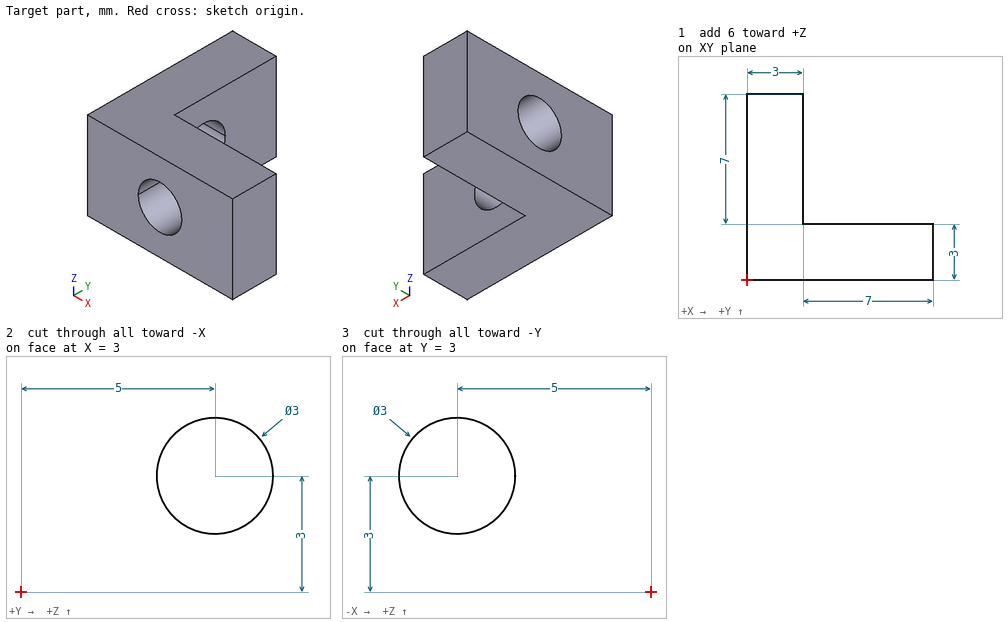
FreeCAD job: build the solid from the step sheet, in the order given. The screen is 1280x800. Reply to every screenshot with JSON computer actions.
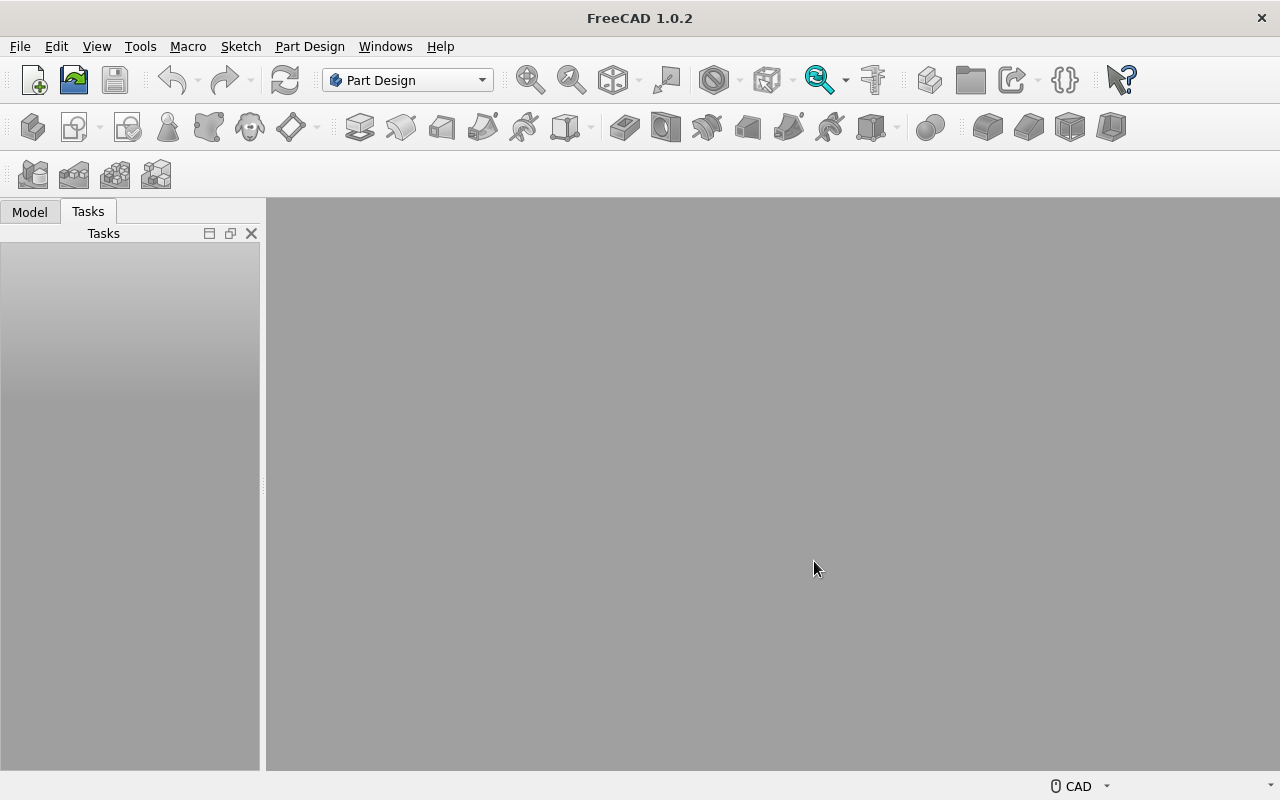
{"action": "left_click", "coordinate": [33, 80]}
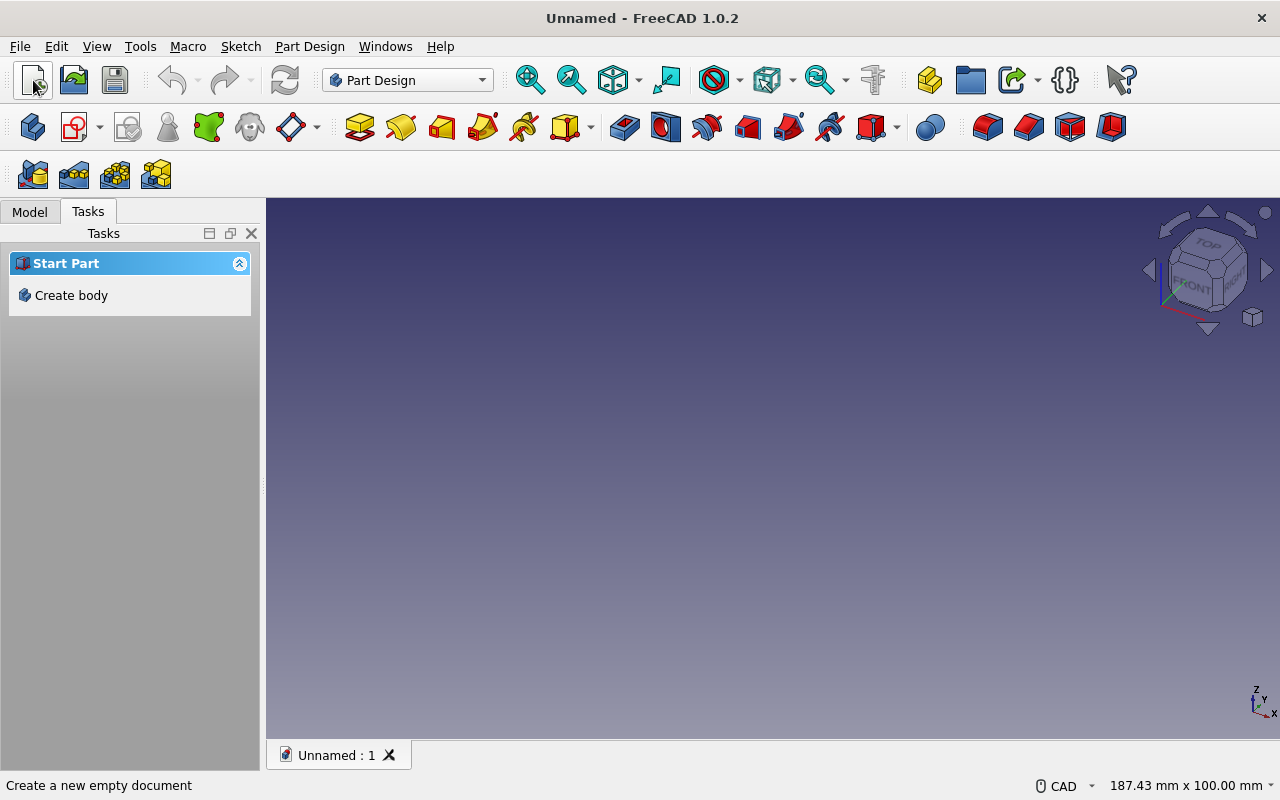
{"action": "left_click", "coordinate": [74, 128]}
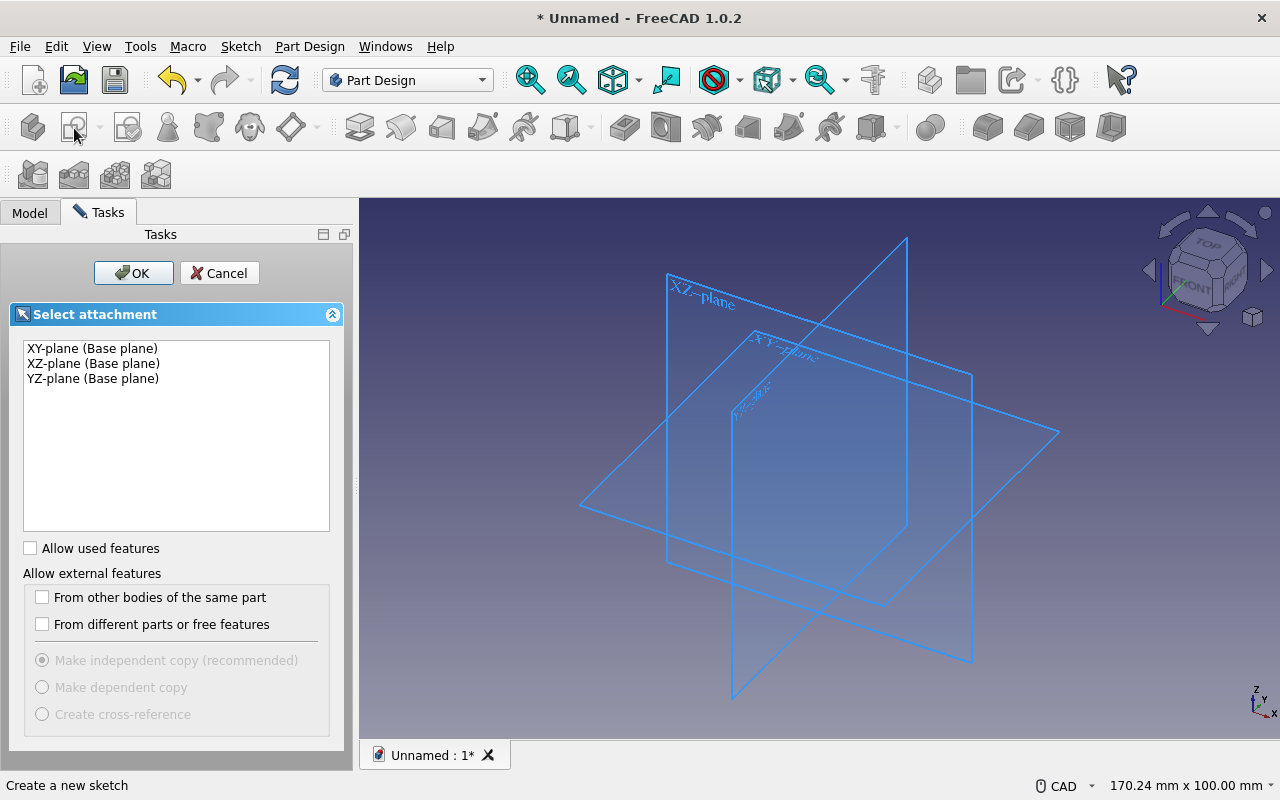
{"action": "left_click", "coordinate": [84, 348]}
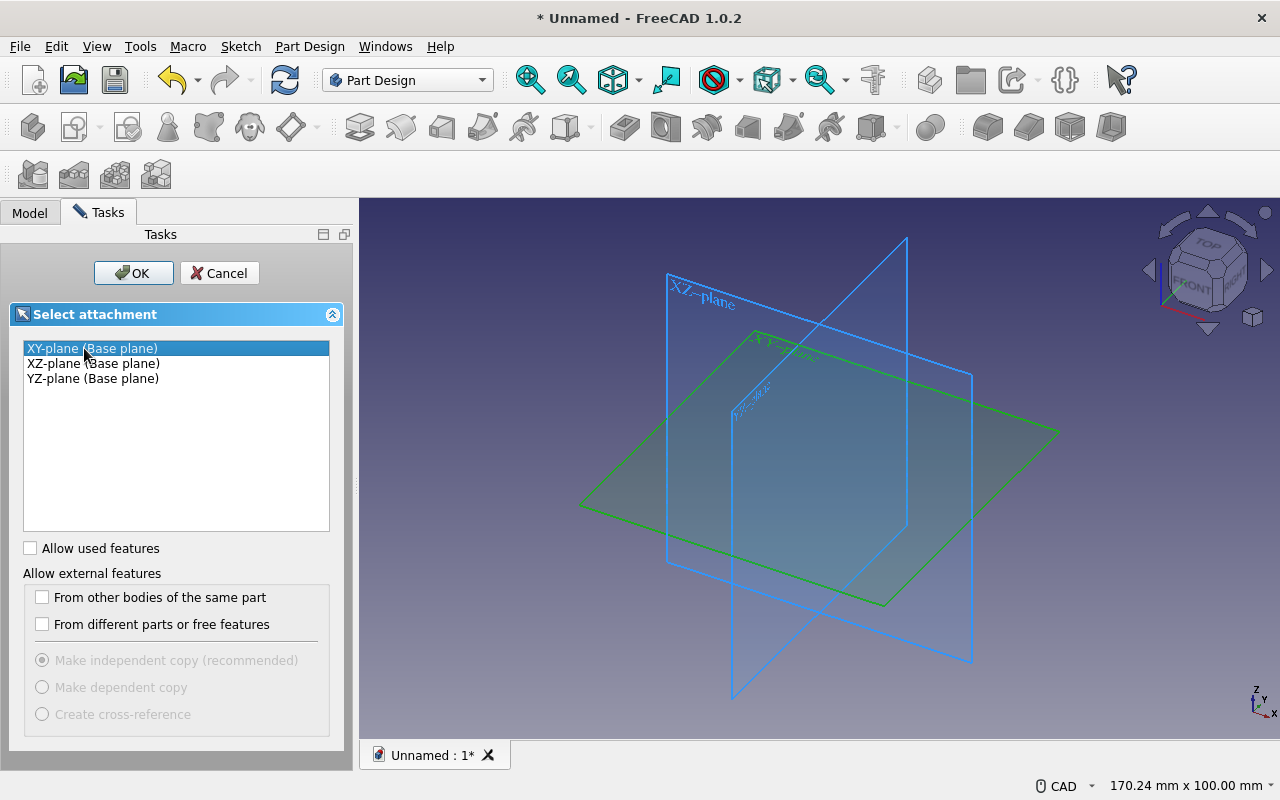
{"action": "left_click", "coordinate": [134, 273]}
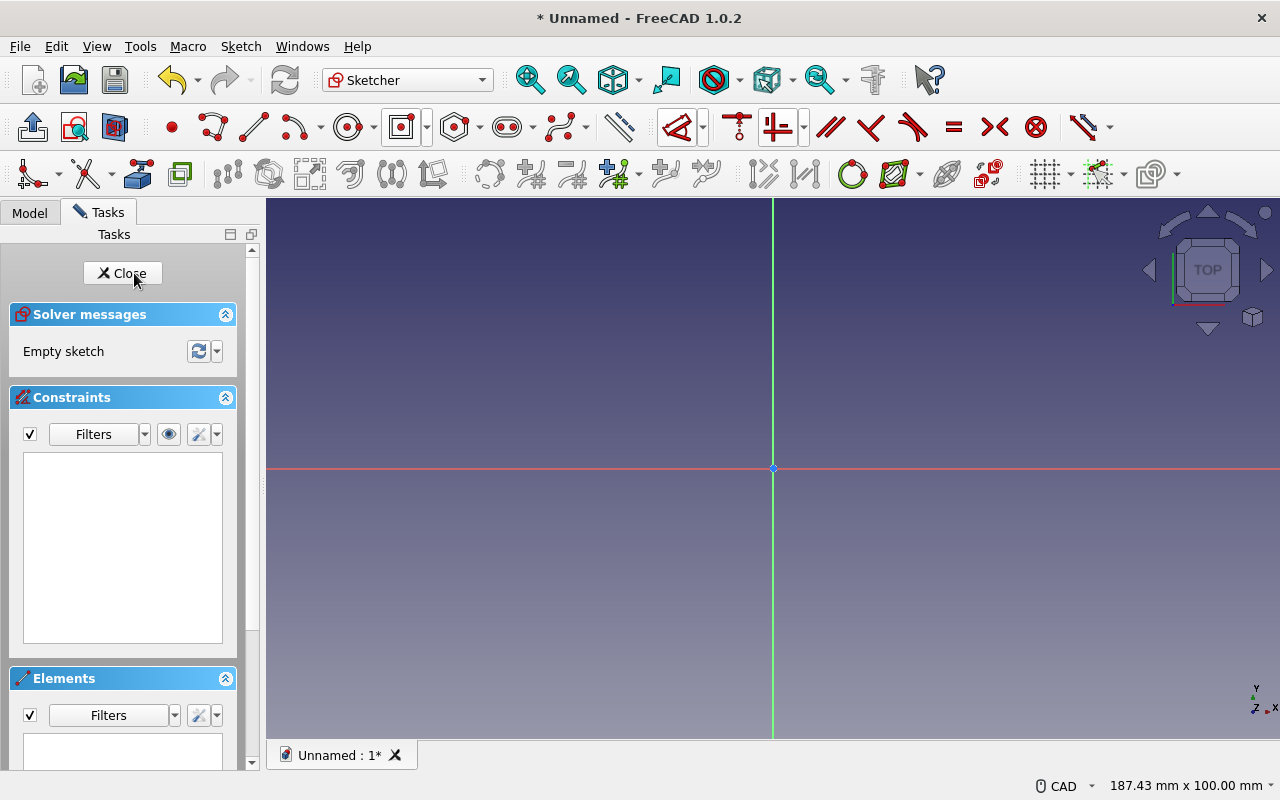
{"action": "scroll", "coordinate": [819, 436], "scroll_direction": "up", "scroll_amount": 9}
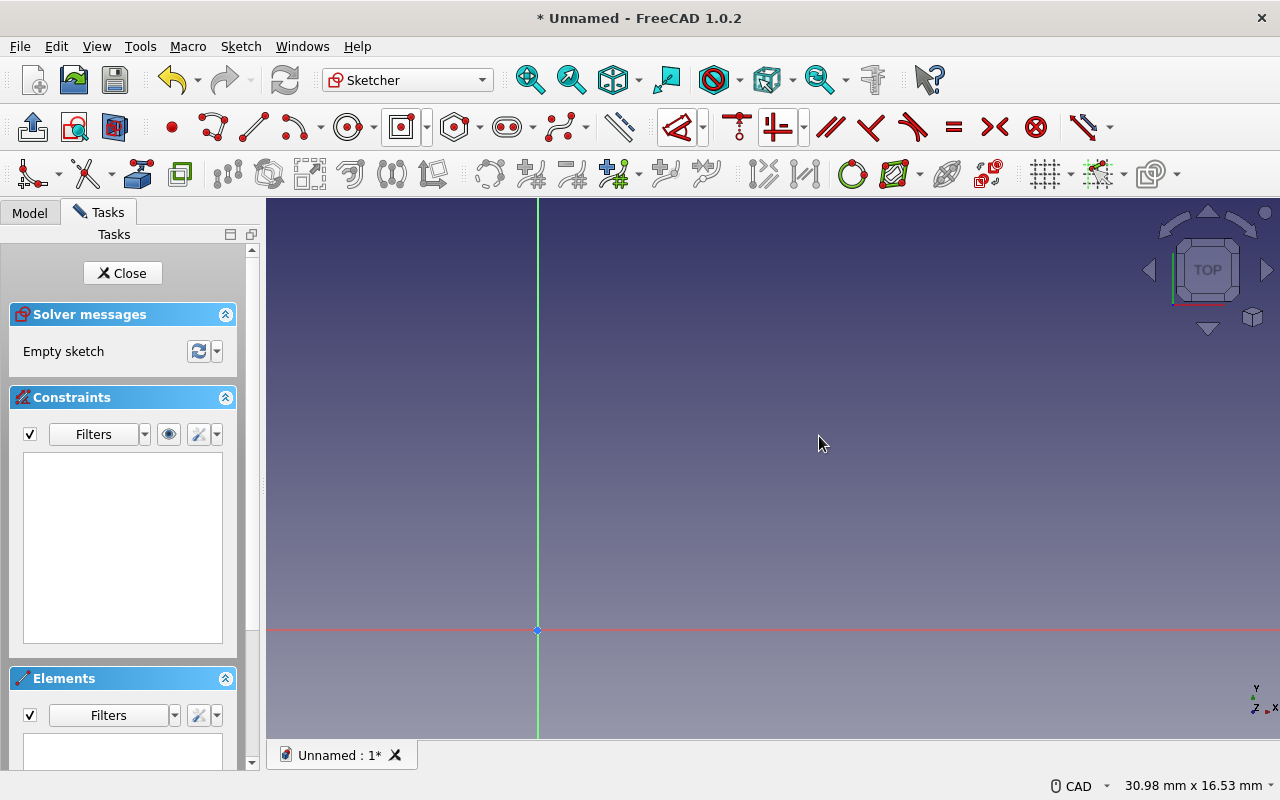
{"action": "left_click", "coordinate": [213, 128]}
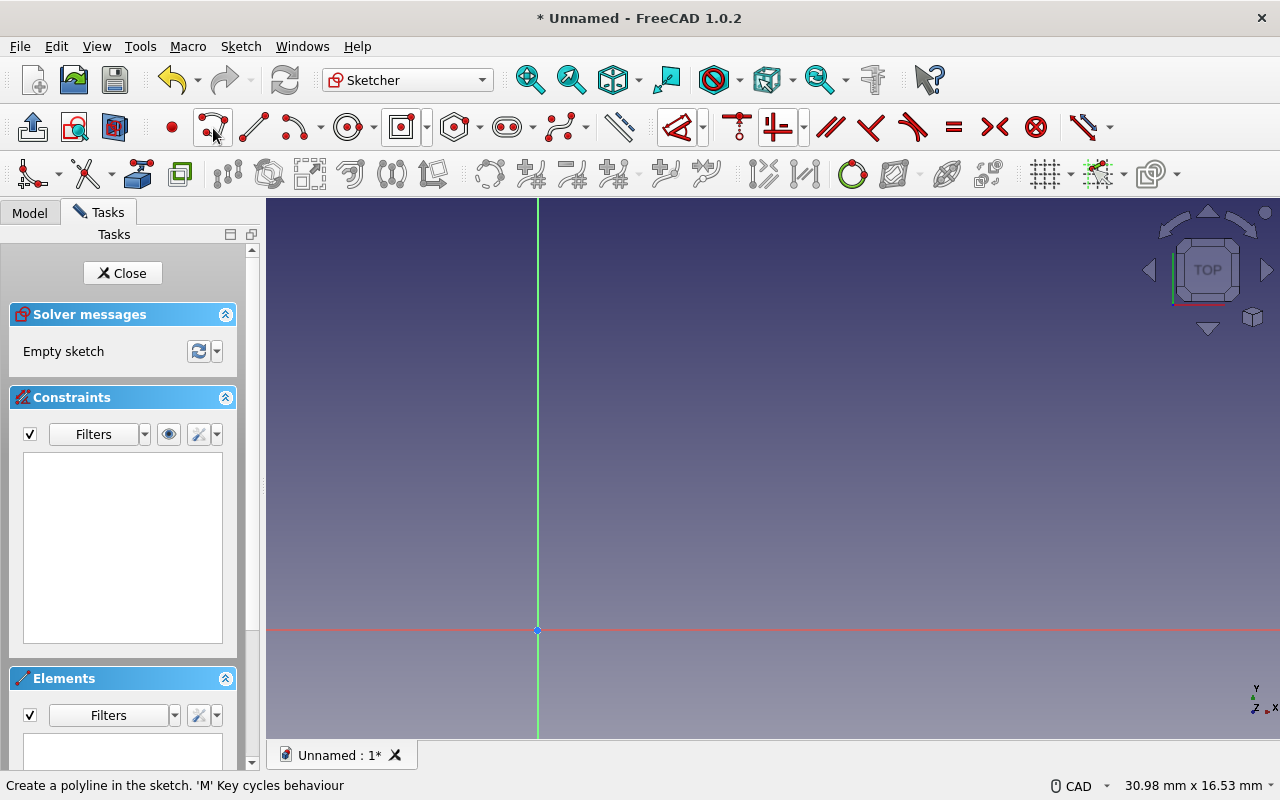
{"action": "left_click", "coordinate": [538, 630]}
{"action": "left_click", "coordinate": [865, 621]}
{"action": "left_click", "coordinate": [865, 532]}
{"action": "left_click", "coordinate": [636, 532]}
{"action": "left_click", "coordinate": [636, 303]}
{"action": "left_click", "coordinate": [547, 303]}
{"action": "left_click", "coordinate": [538, 630]}
{"action": "key", "text": "Escape"}
{"action": "key", "text": "Escape"}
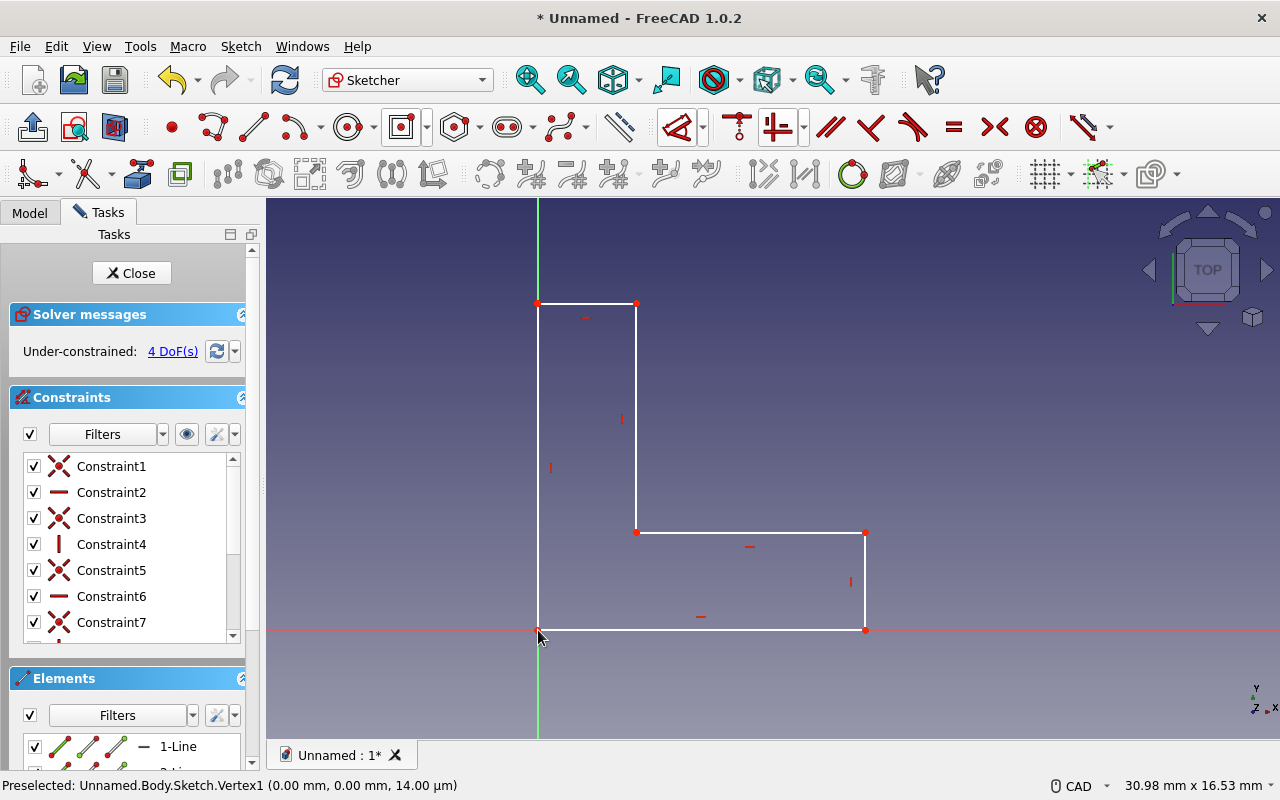
{"action": "left_click", "coordinate": [676, 128]}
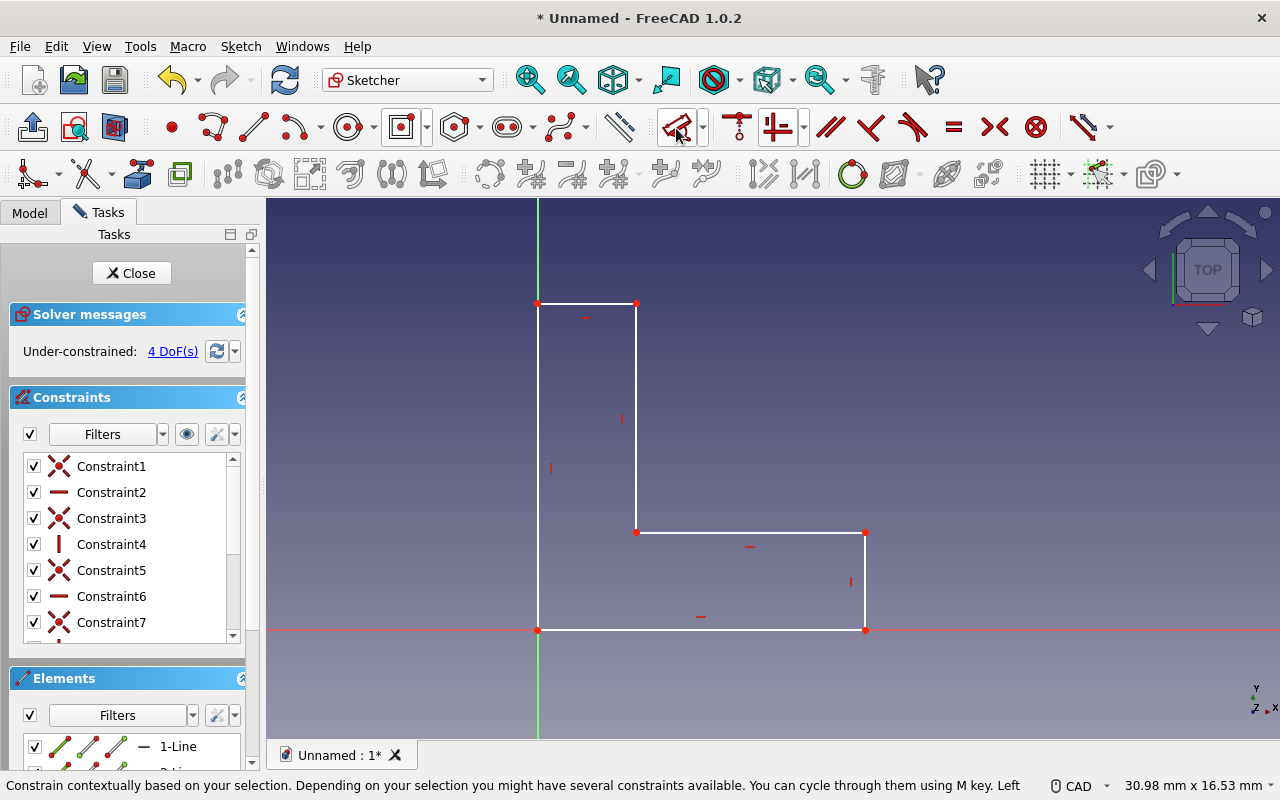
{"action": "left_click", "coordinate": [865, 601]}
{"action": "left_click", "coordinate": [899, 582]}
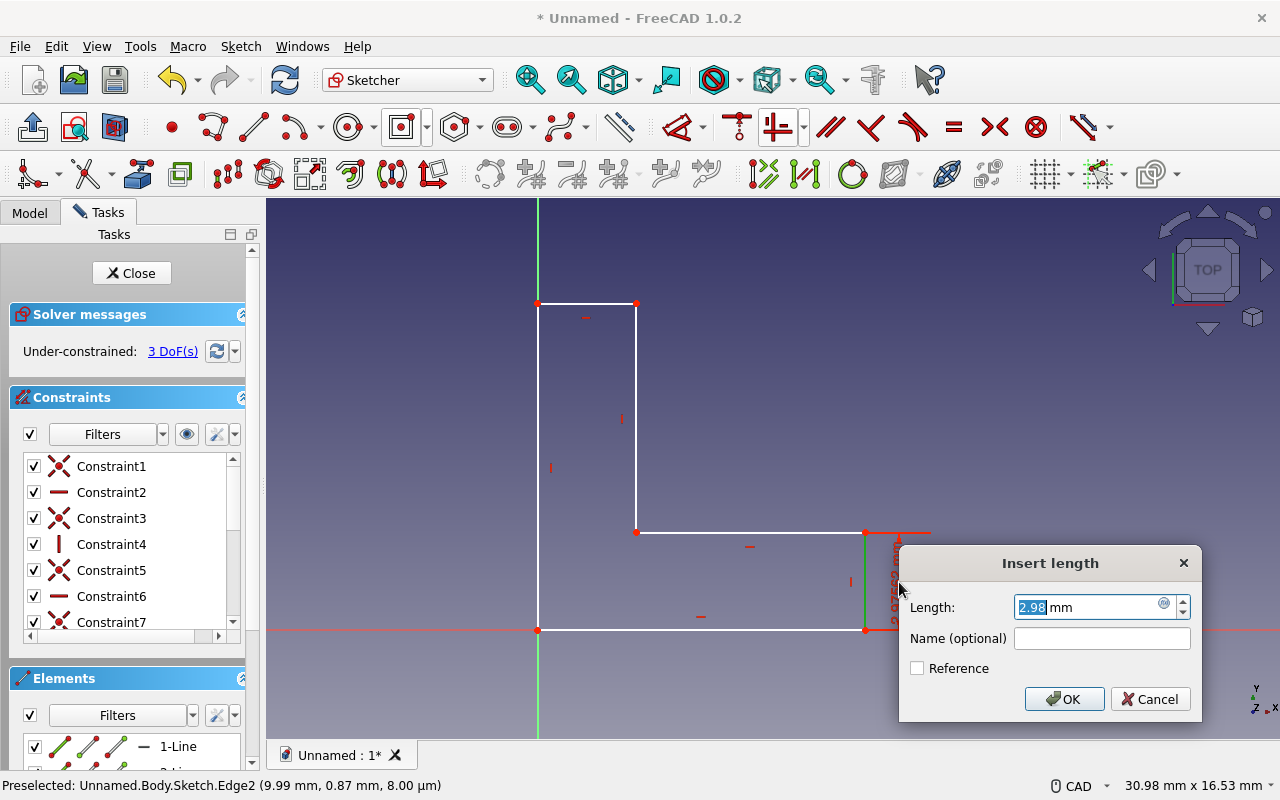
{"action": "type", "text": "3"}
{"action": "key", "text": "Return"}